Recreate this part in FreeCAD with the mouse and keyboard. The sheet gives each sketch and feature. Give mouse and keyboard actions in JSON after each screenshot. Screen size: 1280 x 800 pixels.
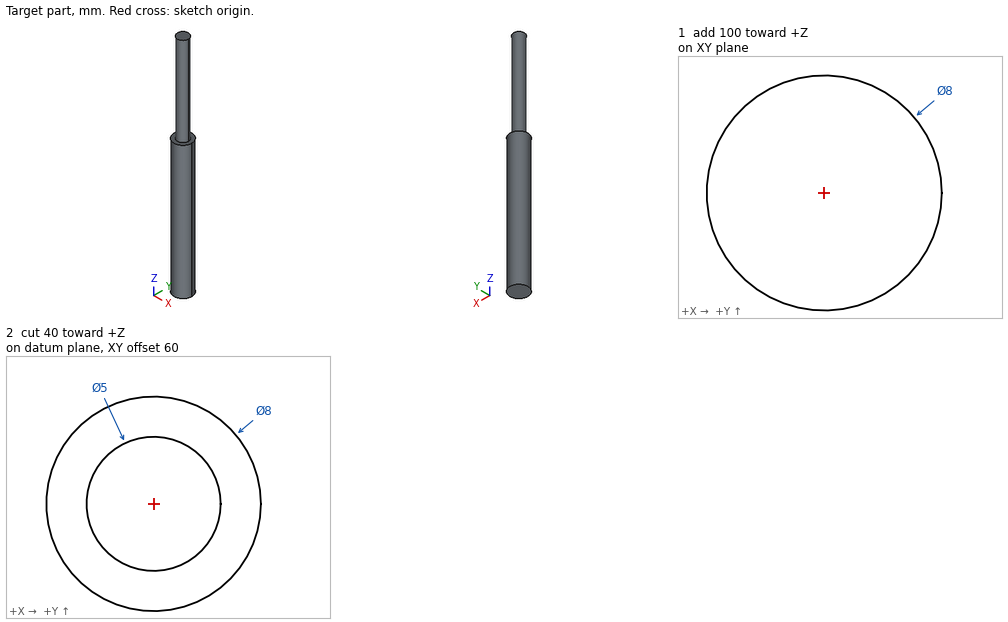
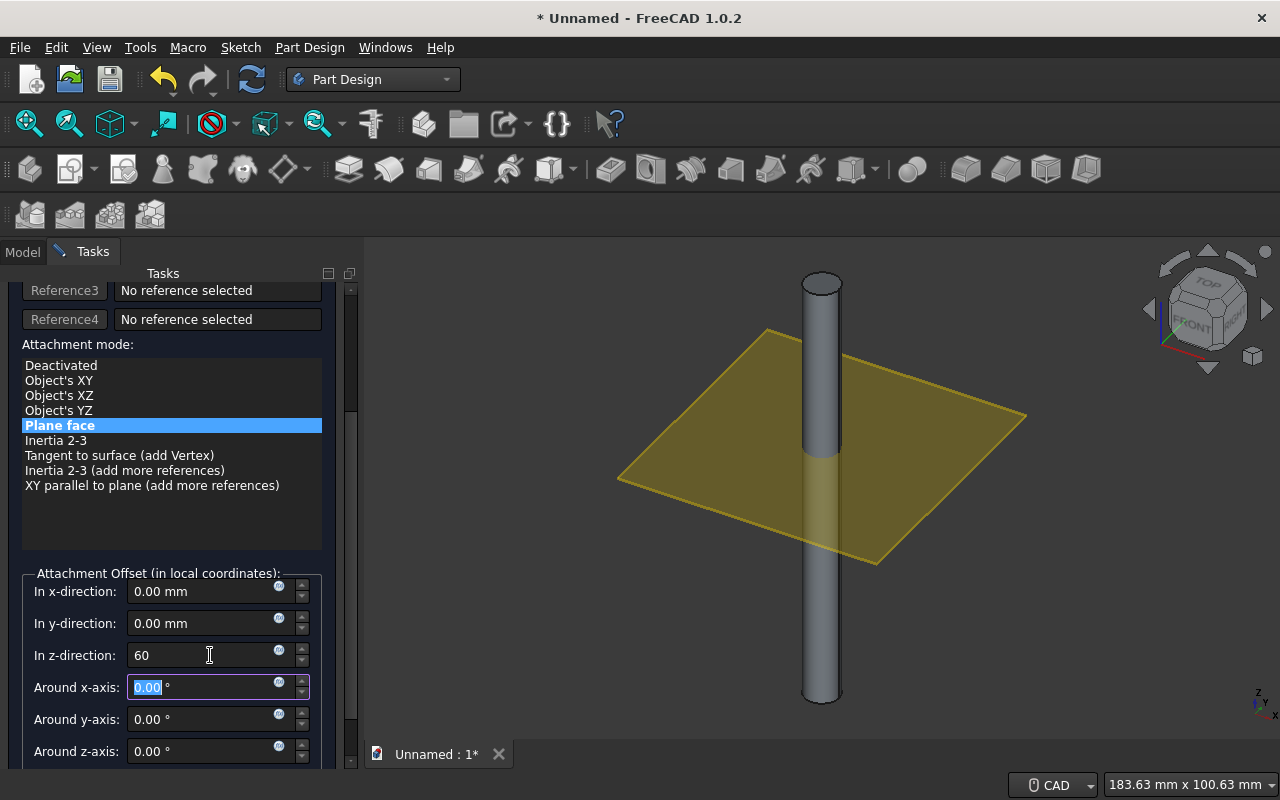
{"action": "scroll", "coordinate": [351, 526], "scroll_direction": "up", "scroll_amount": 4}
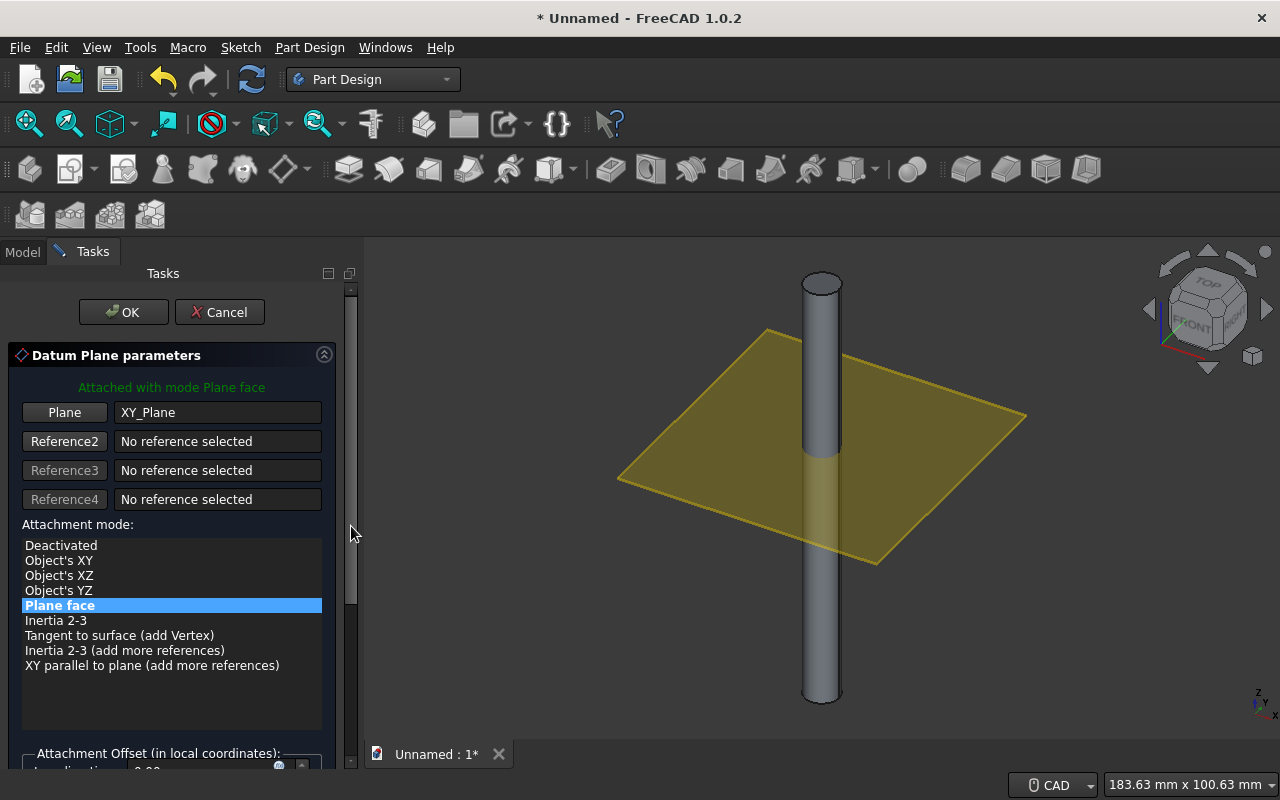
{"action": "left_click", "coordinate": [124, 312]}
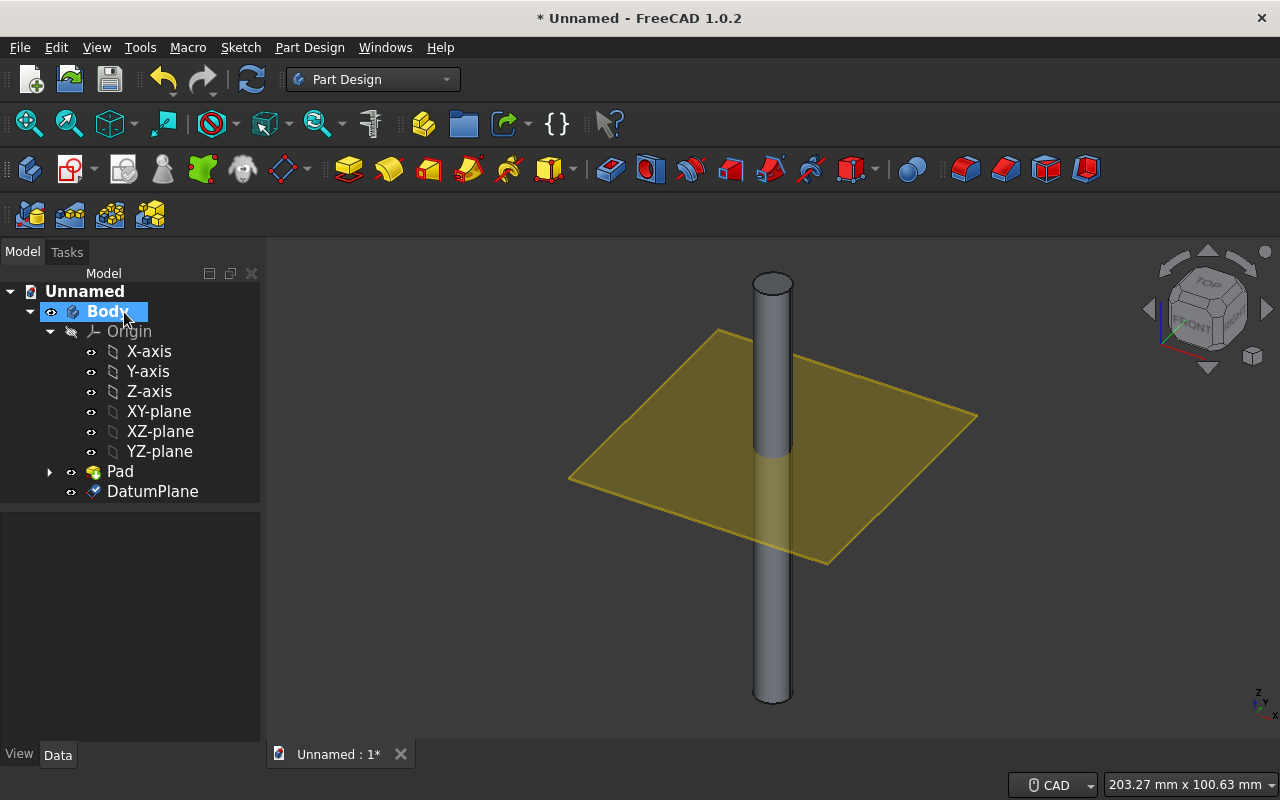
{"action": "left_click", "coordinate": [116, 492]}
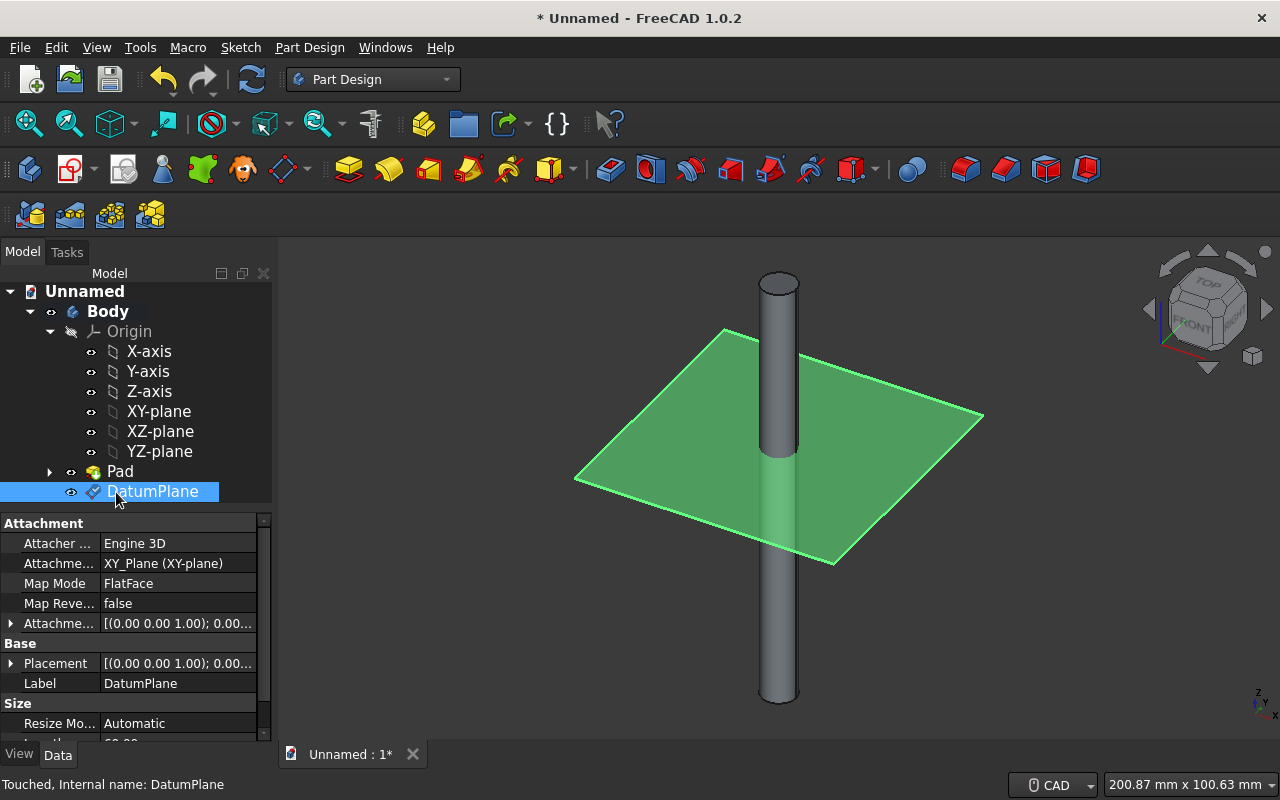
{"action": "left_click", "coordinate": [70, 170]}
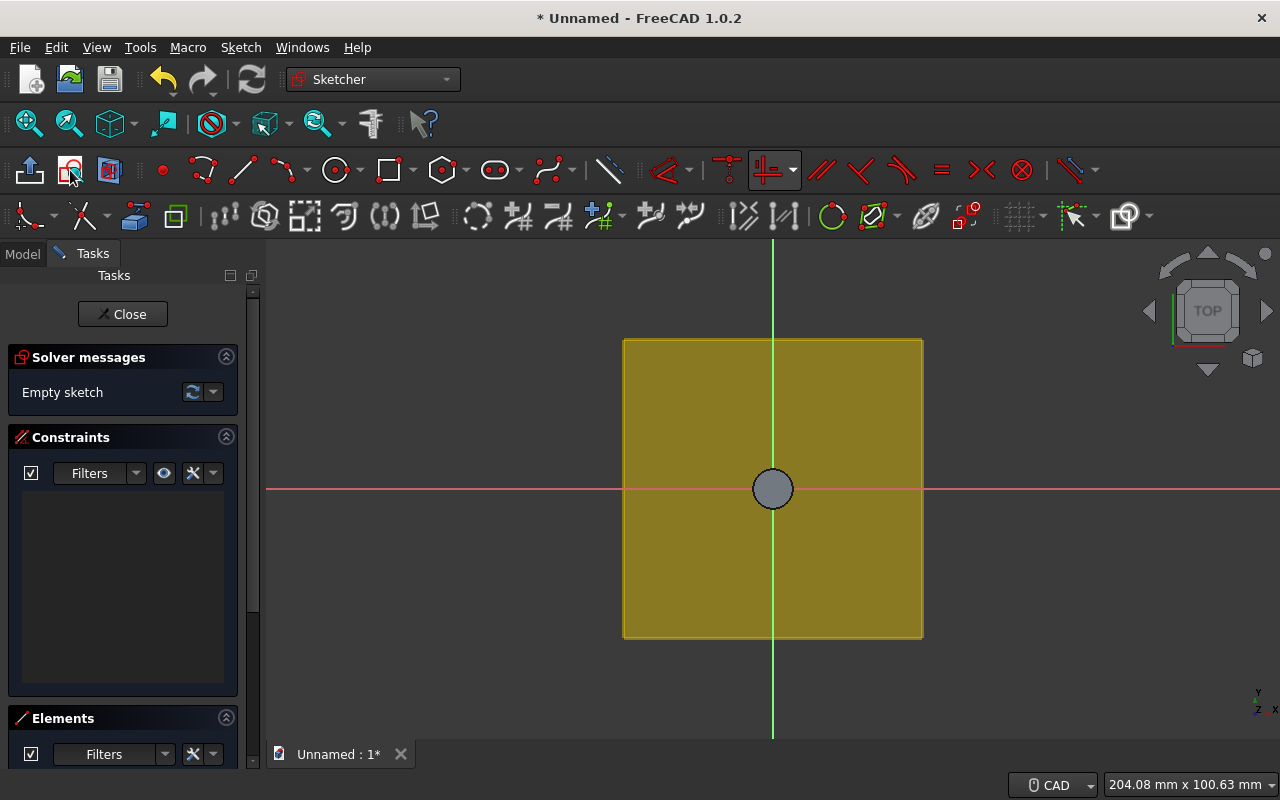
{"action": "key", "text": "q s"}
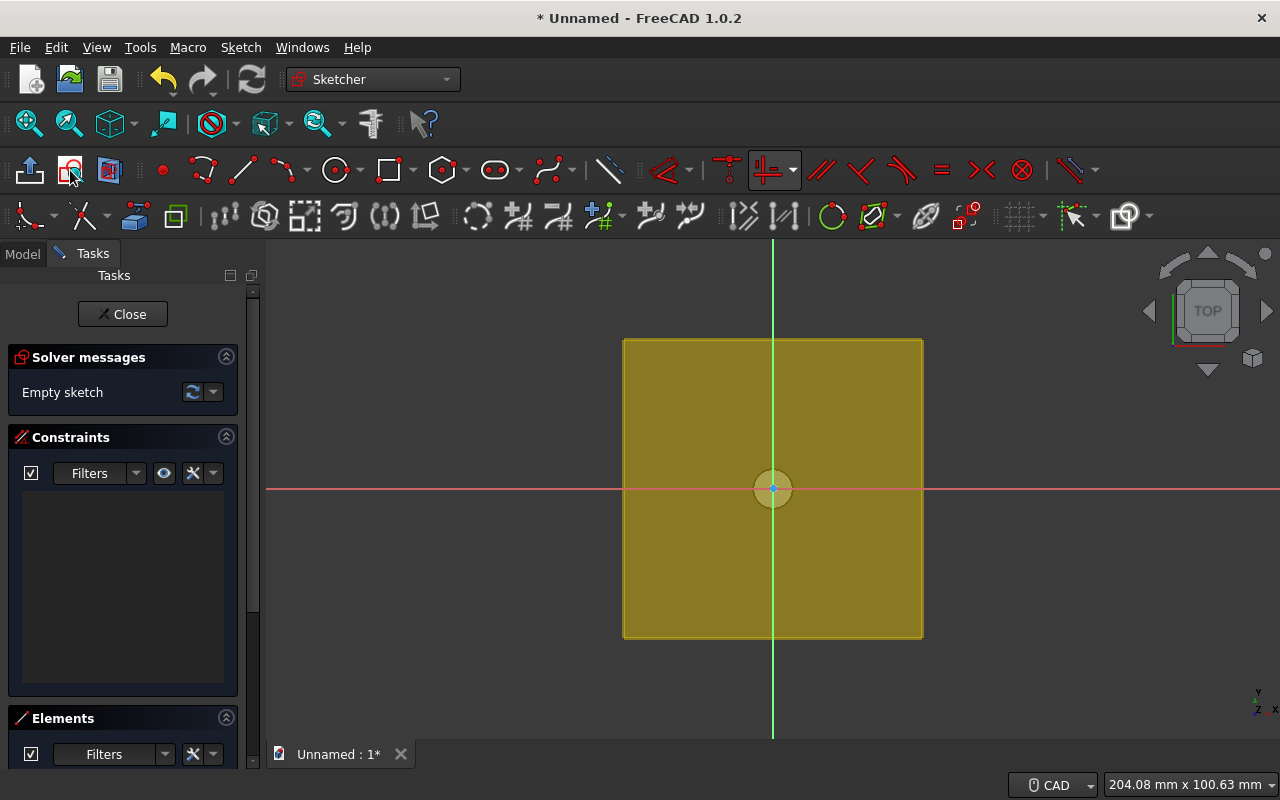
{"action": "scroll", "coordinate": [784, 489], "scroll_direction": "up", "scroll_amount": 10}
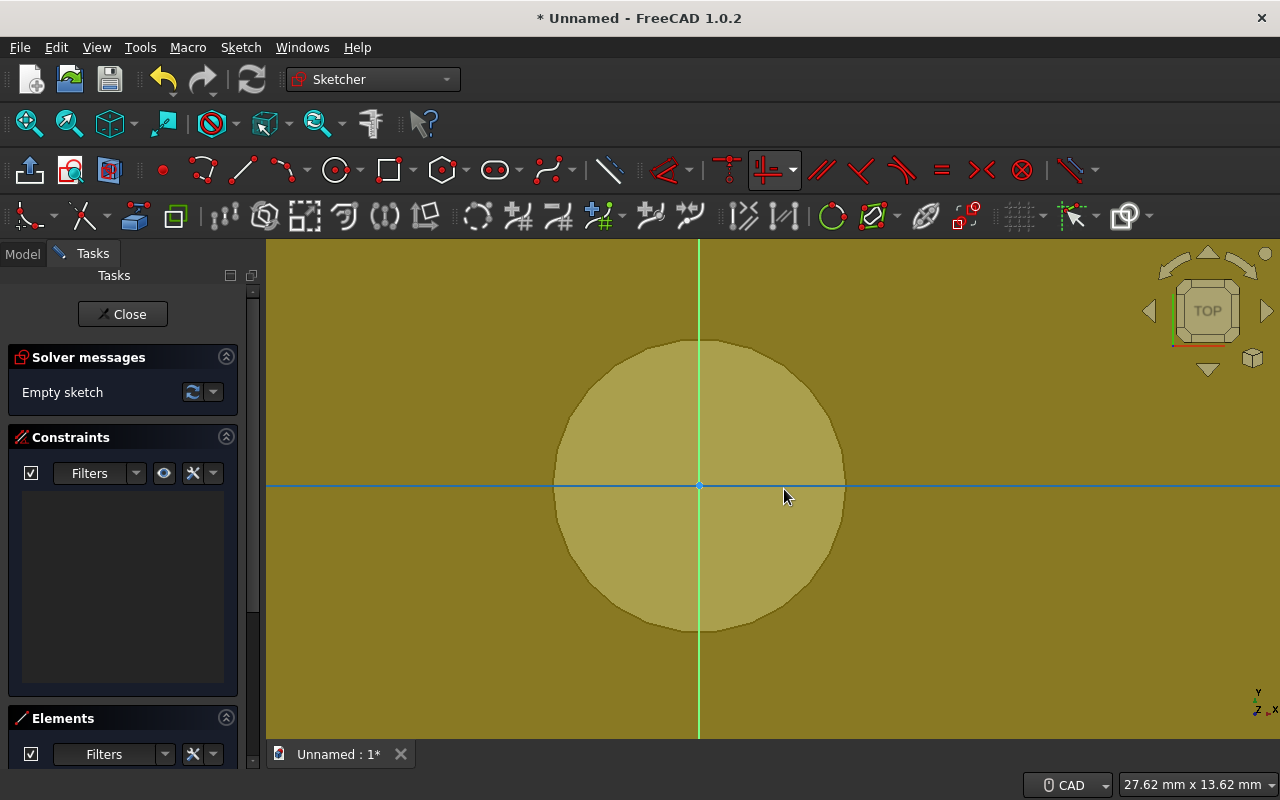
{"action": "left_click", "coordinate": [336, 170]}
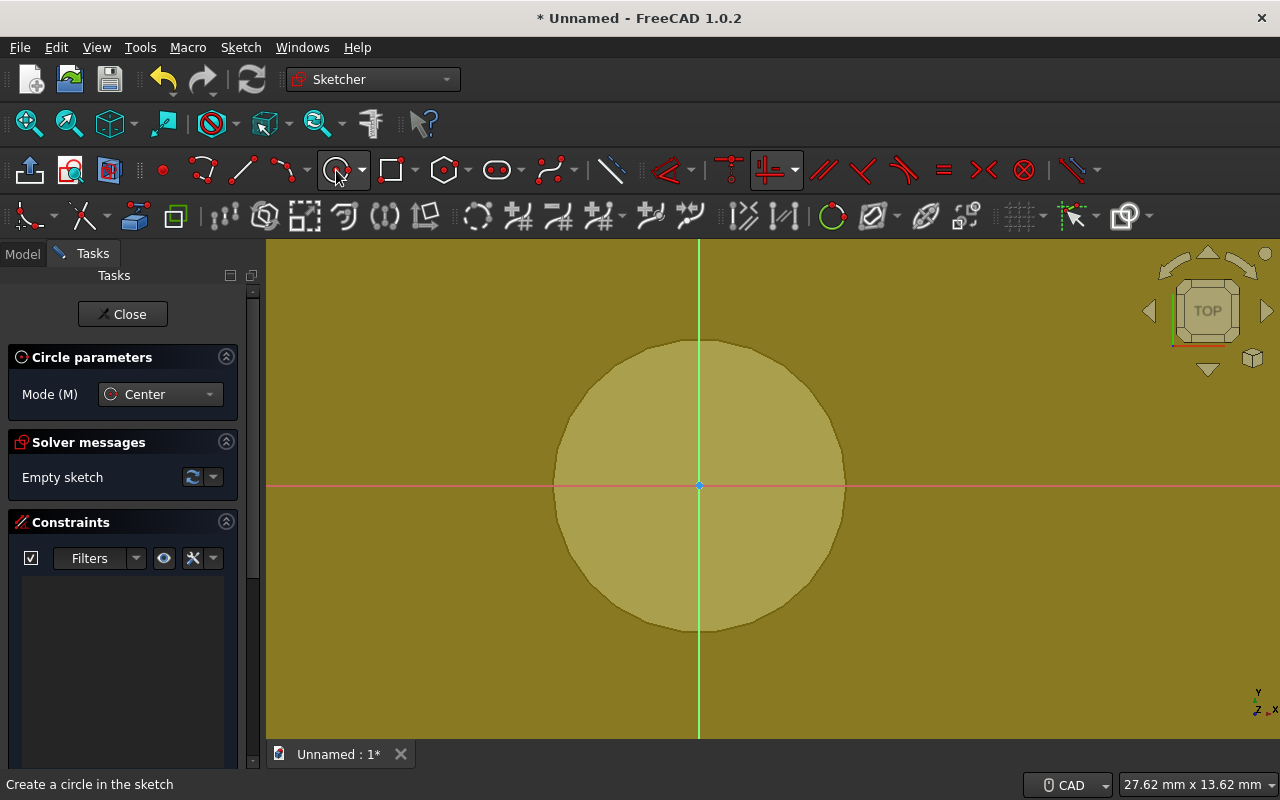
{"action": "left_click", "coordinate": [699, 486]}
{"action": "mouse_move", "coordinate": [803, 382]}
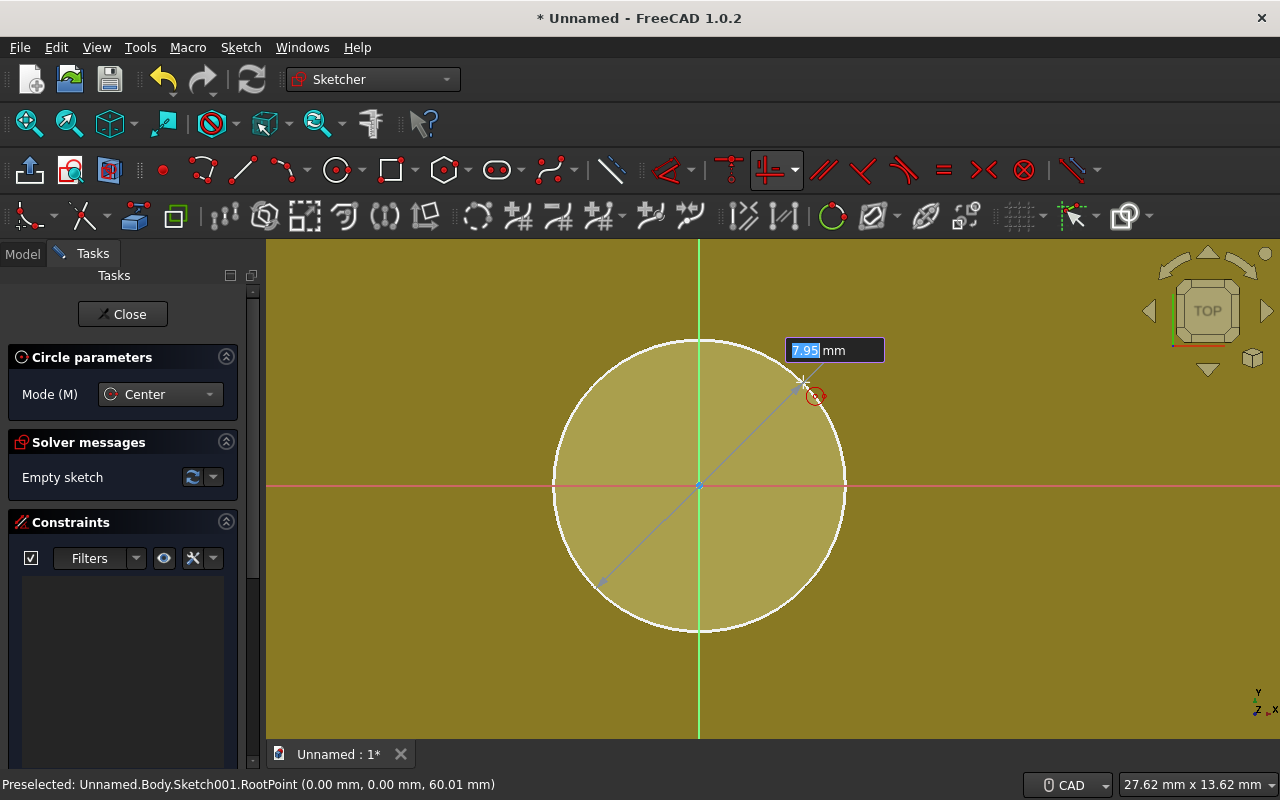
{"action": "type", "text": "8"}
{"action": "key", "text": "Return"}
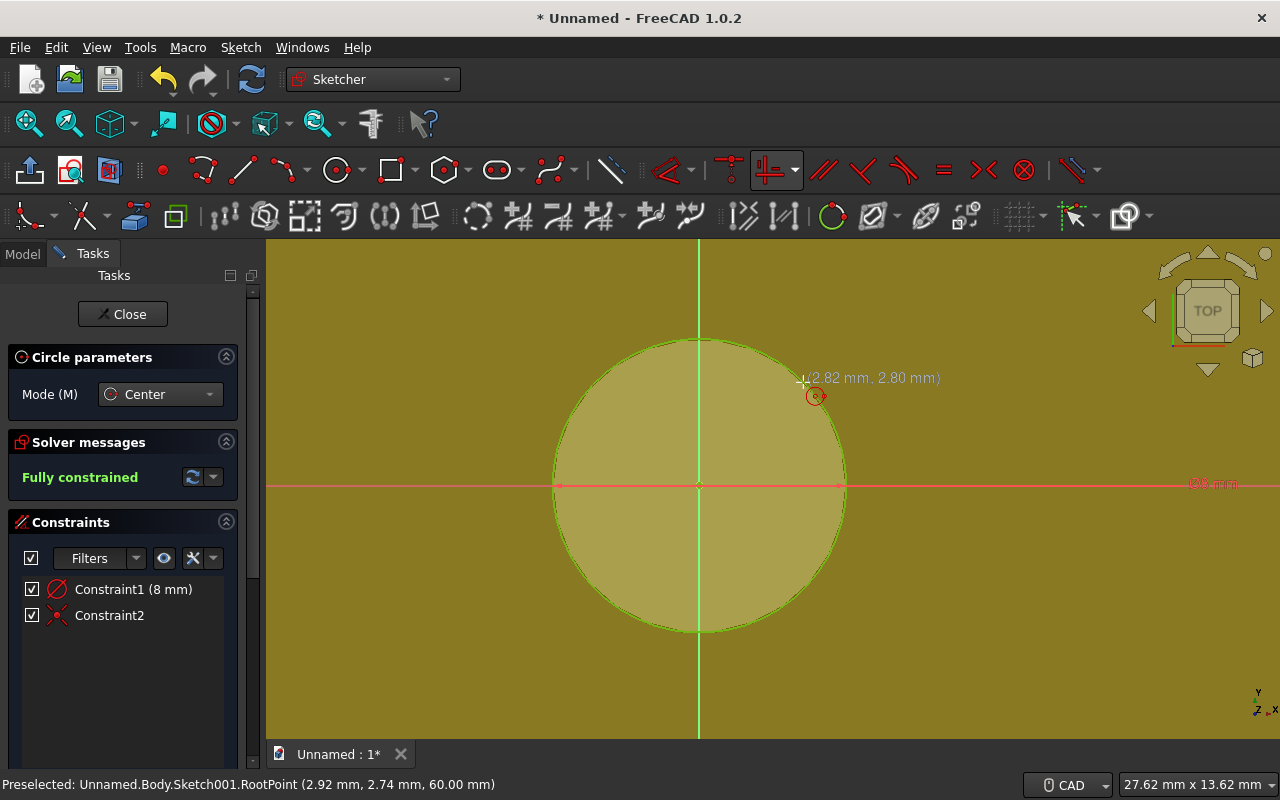
{"action": "left_click", "coordinate": [699, 486]}
{"action": "mouse_move", "coordinate": [764, 421]}